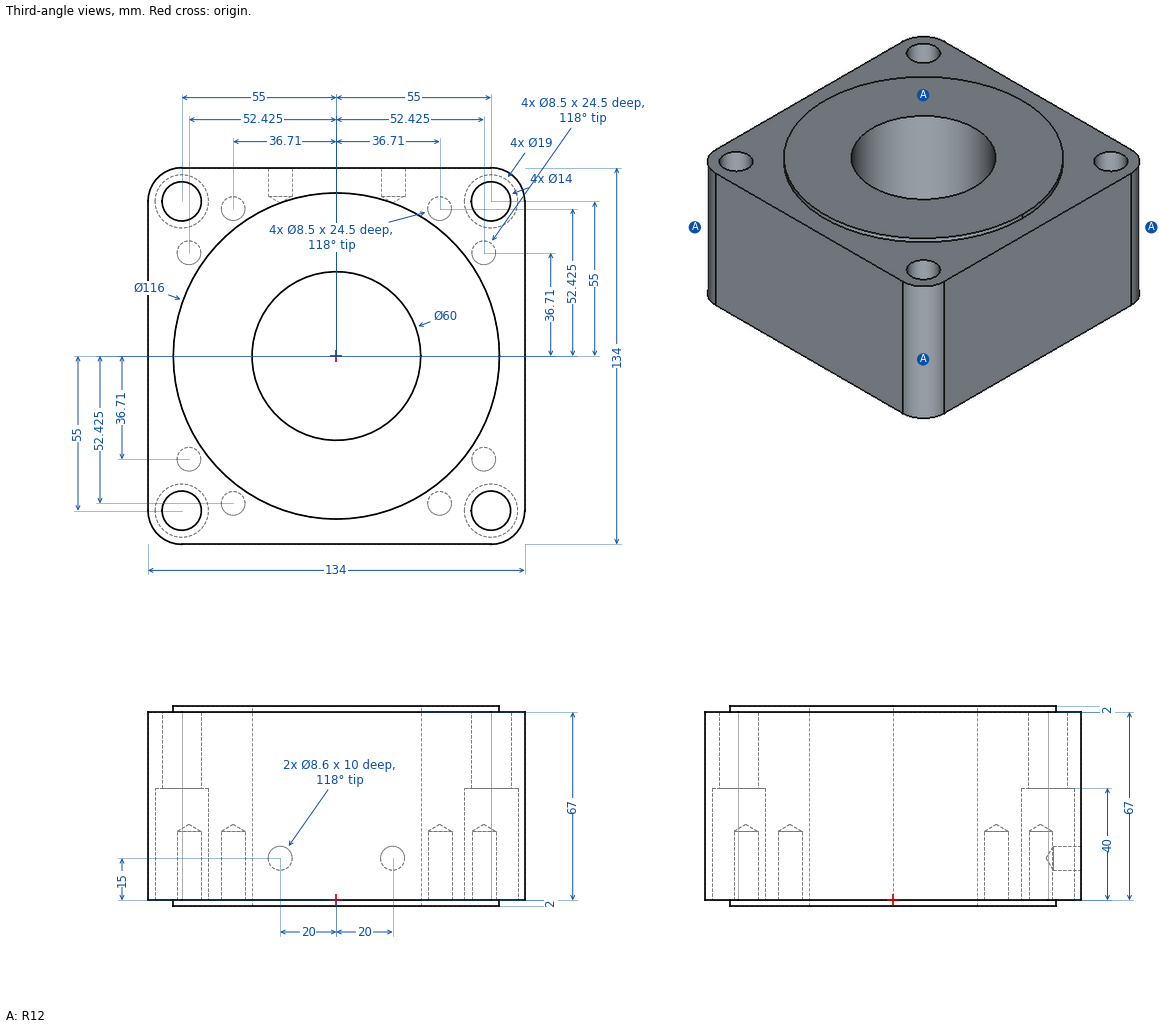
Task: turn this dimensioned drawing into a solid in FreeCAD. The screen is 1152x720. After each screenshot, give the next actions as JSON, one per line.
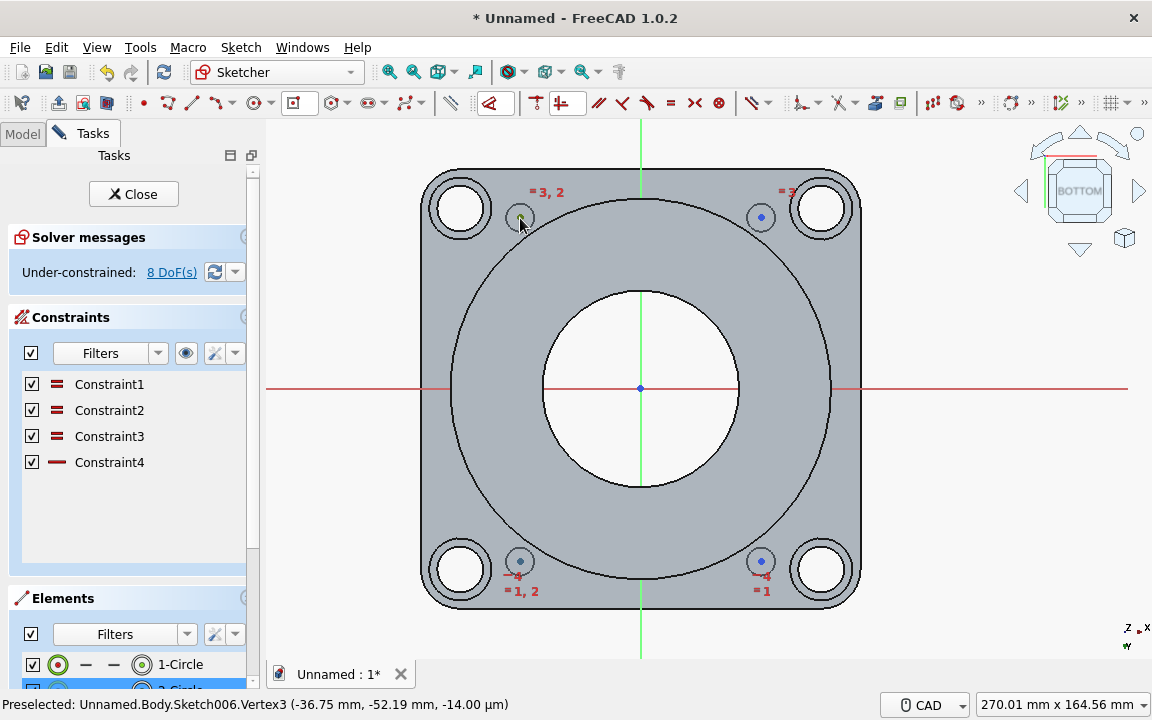
{"action": "key", "text": "v"}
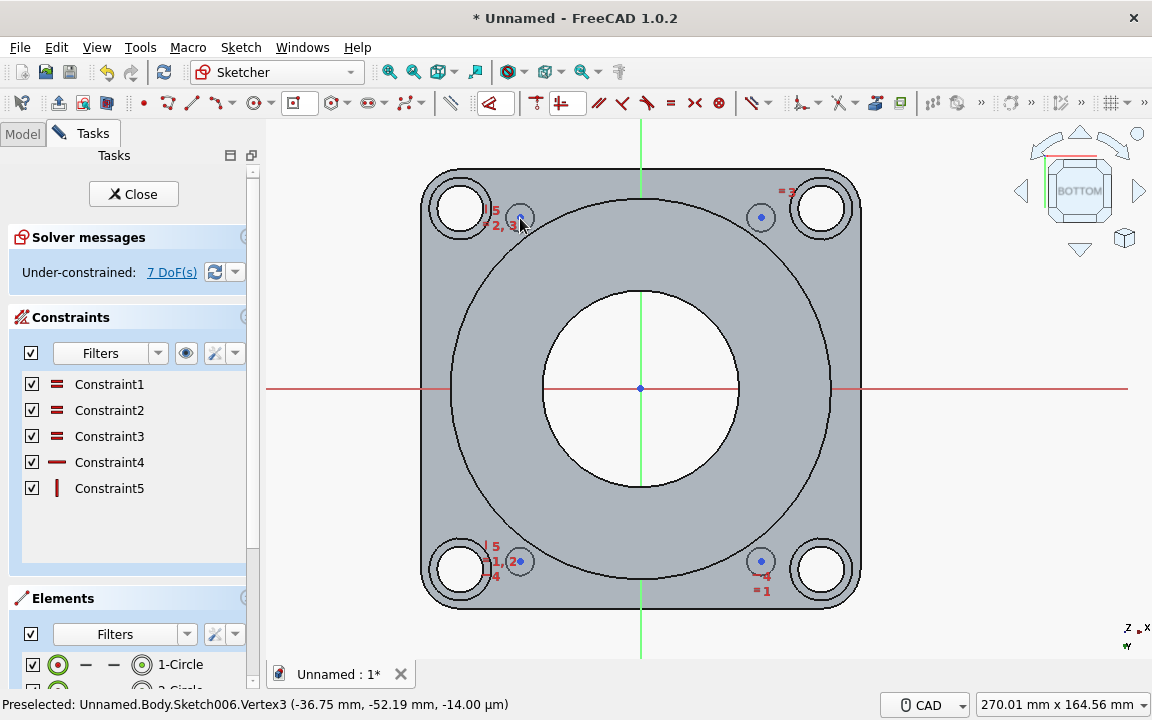
{"action": "left_click", "coordinate": [761, 562]}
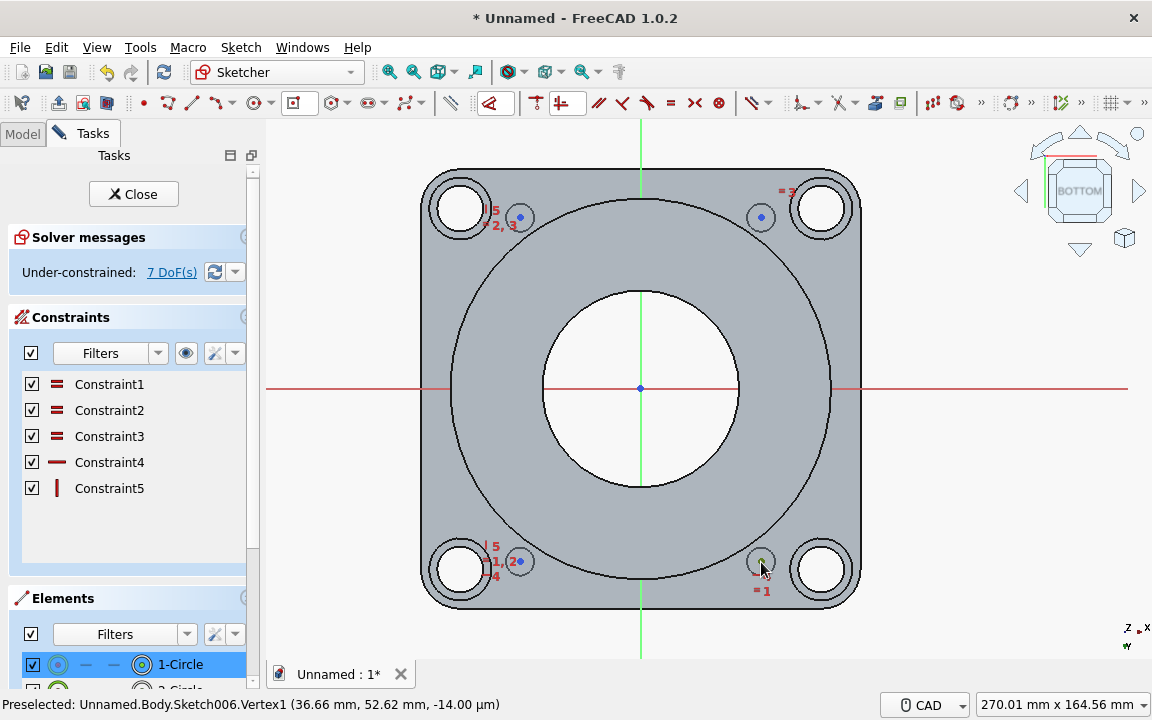
{"action": "left_click", "coordinate": [761, 218]}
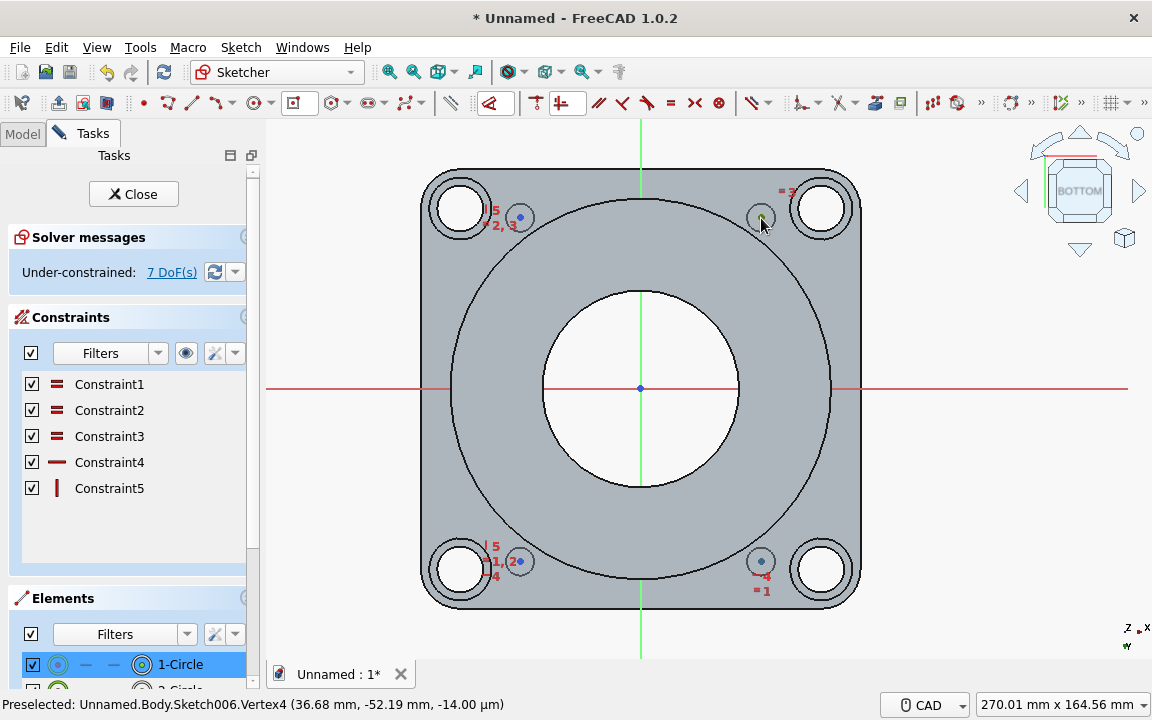
{"action": "key", "text": "v"}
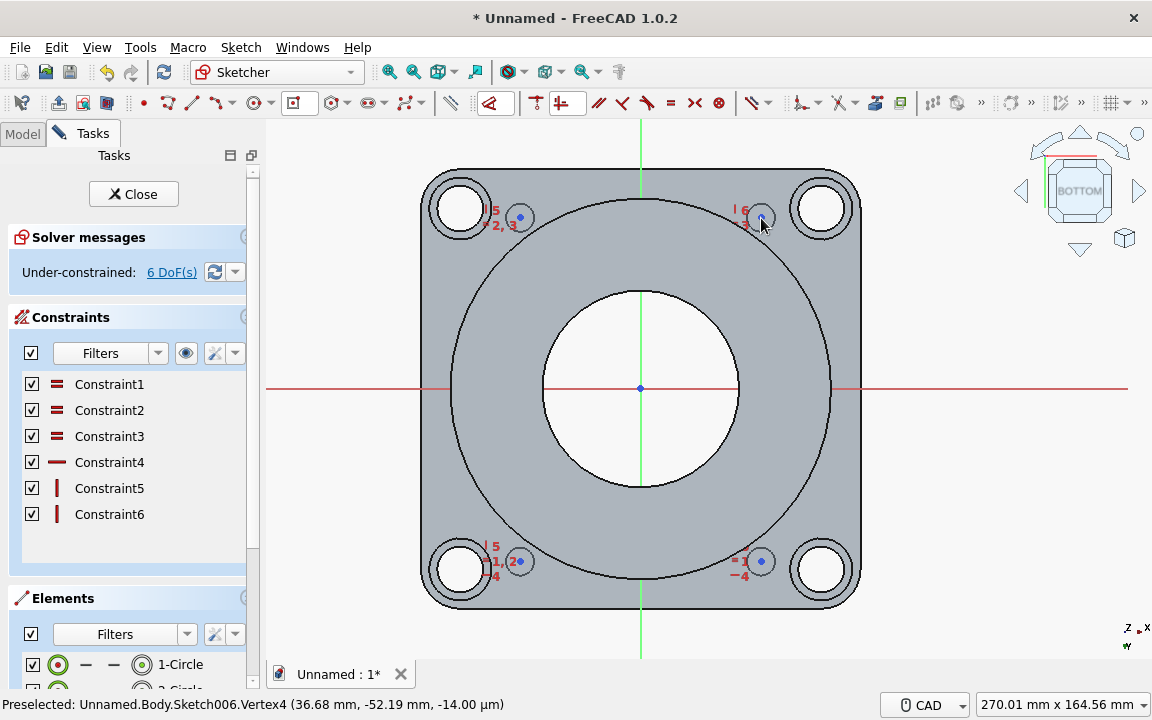
{"action": "left_click", "coordinate": [520, 218]}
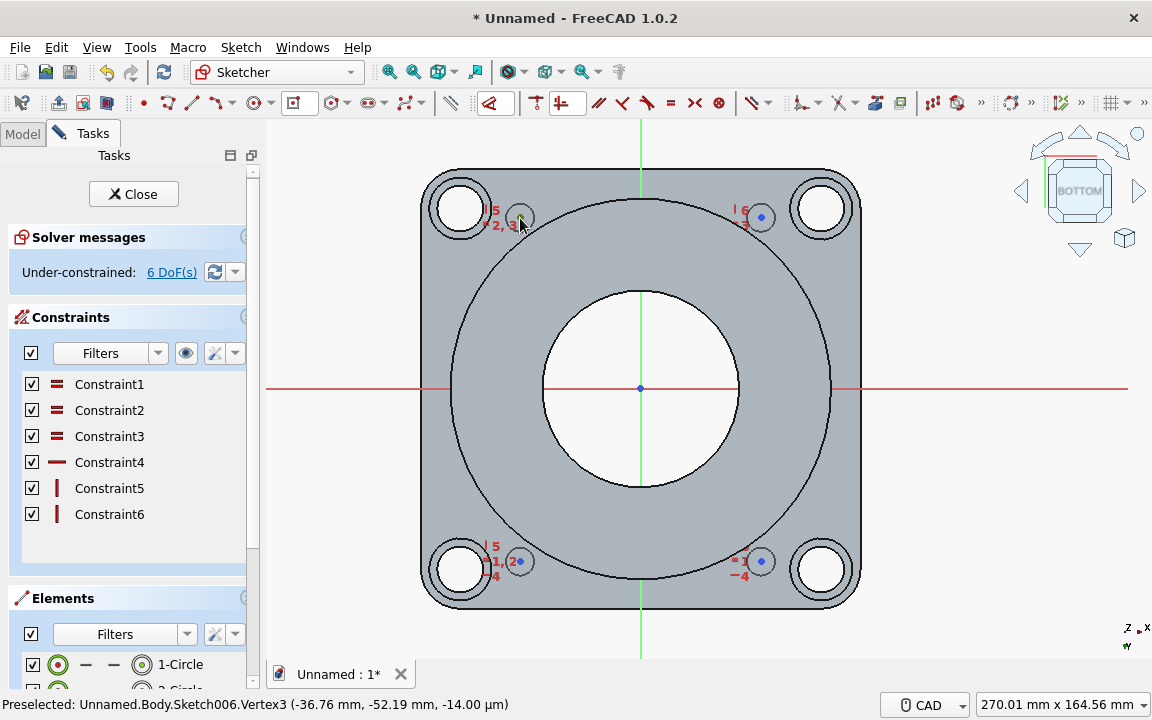
{"action": "left_click", "coordinate": [761, 218]}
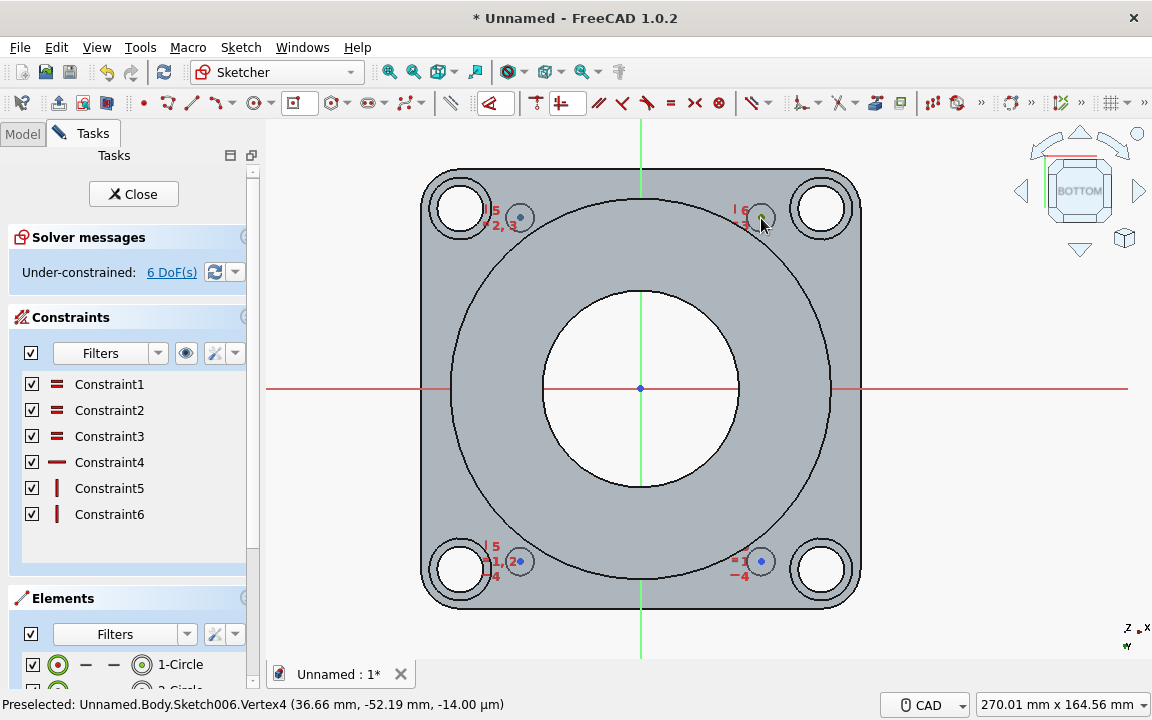
{"action": "key", "text": "h"}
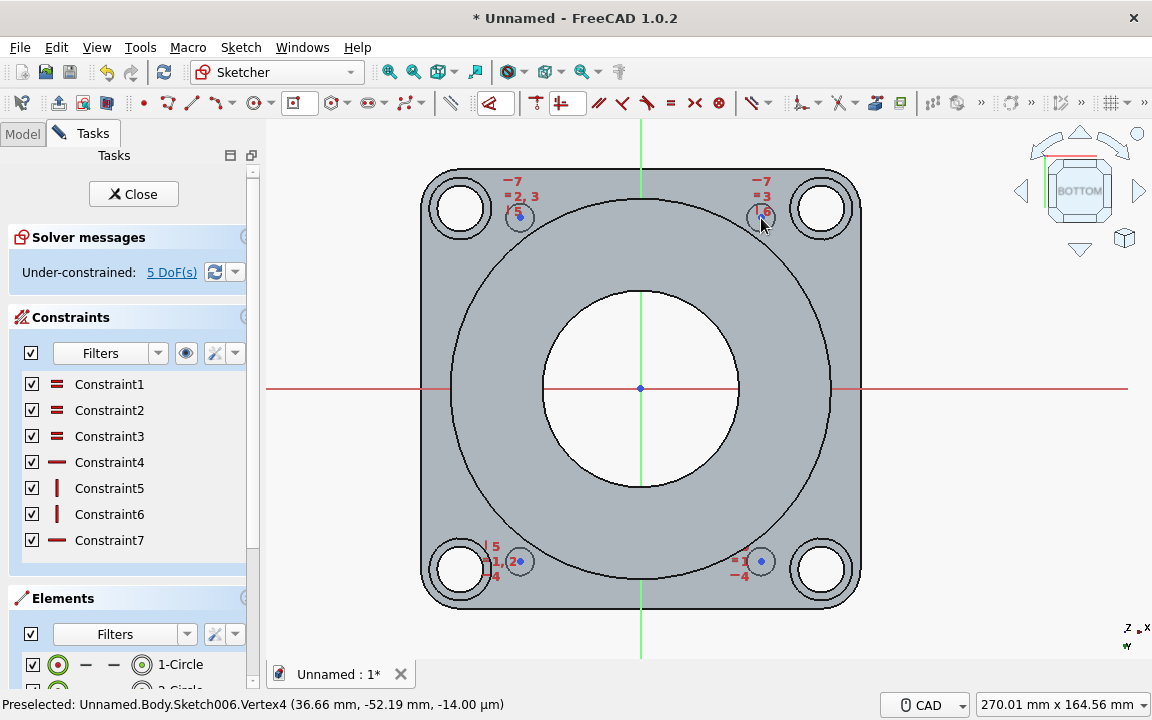
{"action": "scroll", "coordinate": [771, 552], "scroll_direction": "up", "scroll_amount": 2}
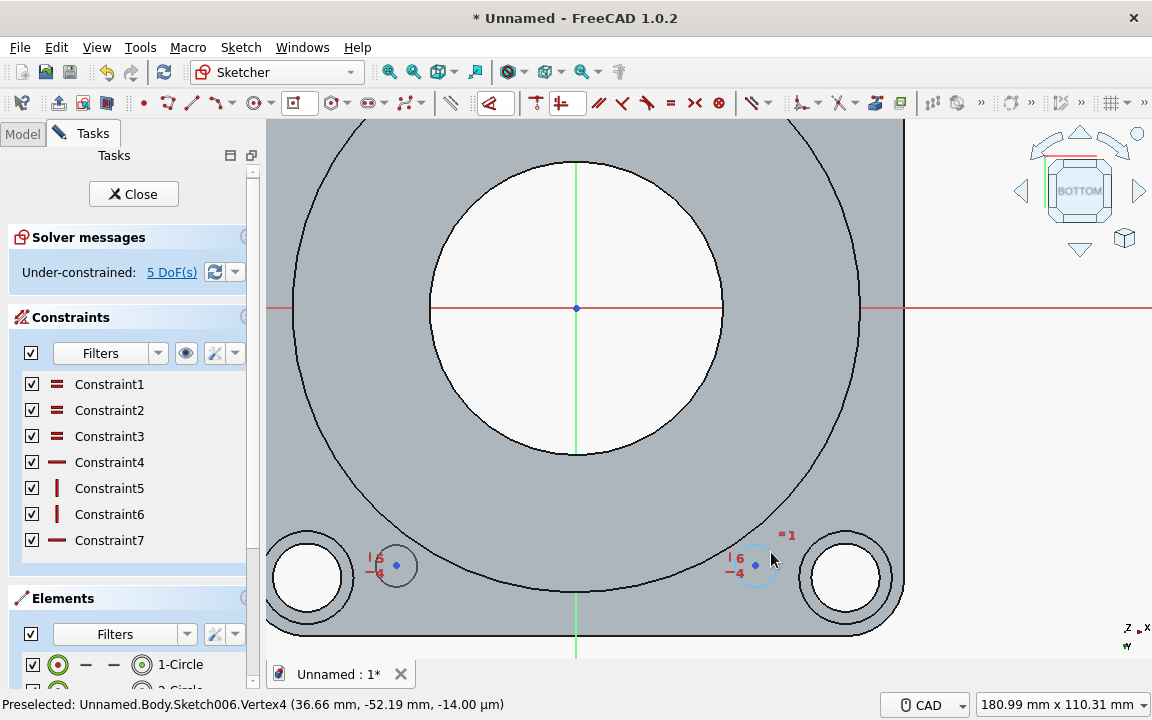
{"action": "left_click", "coordinate": [771, 551]}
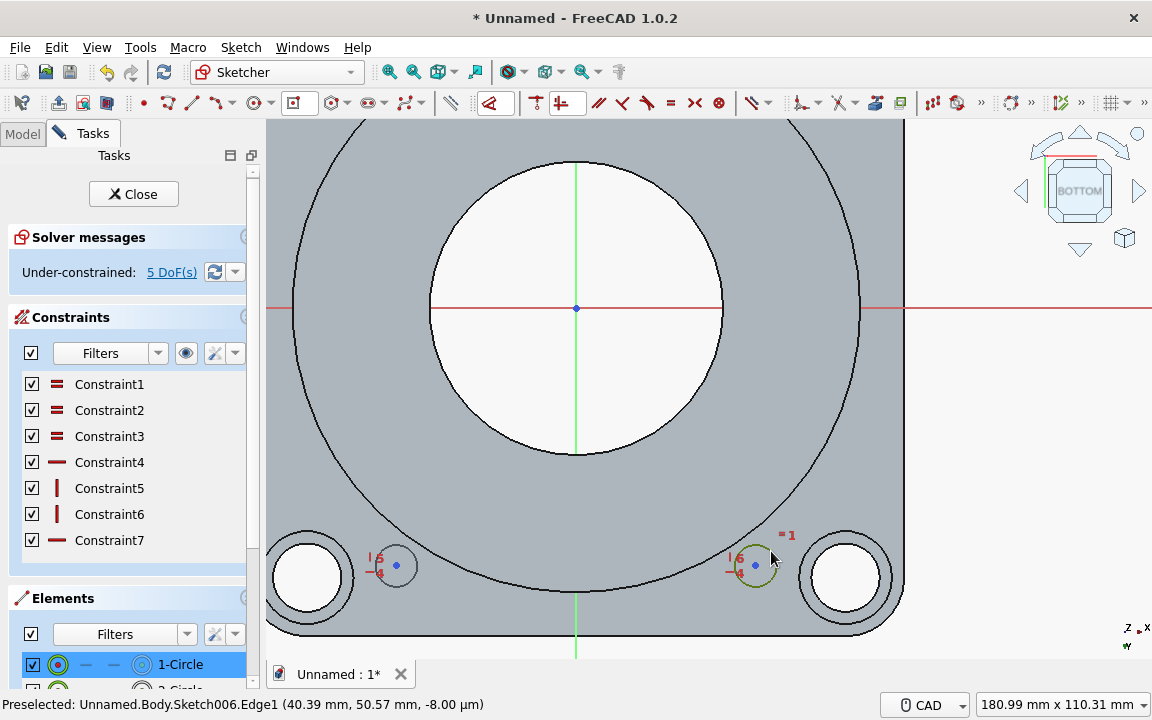
{"action": "left_click", "coordinate": [508, 104]}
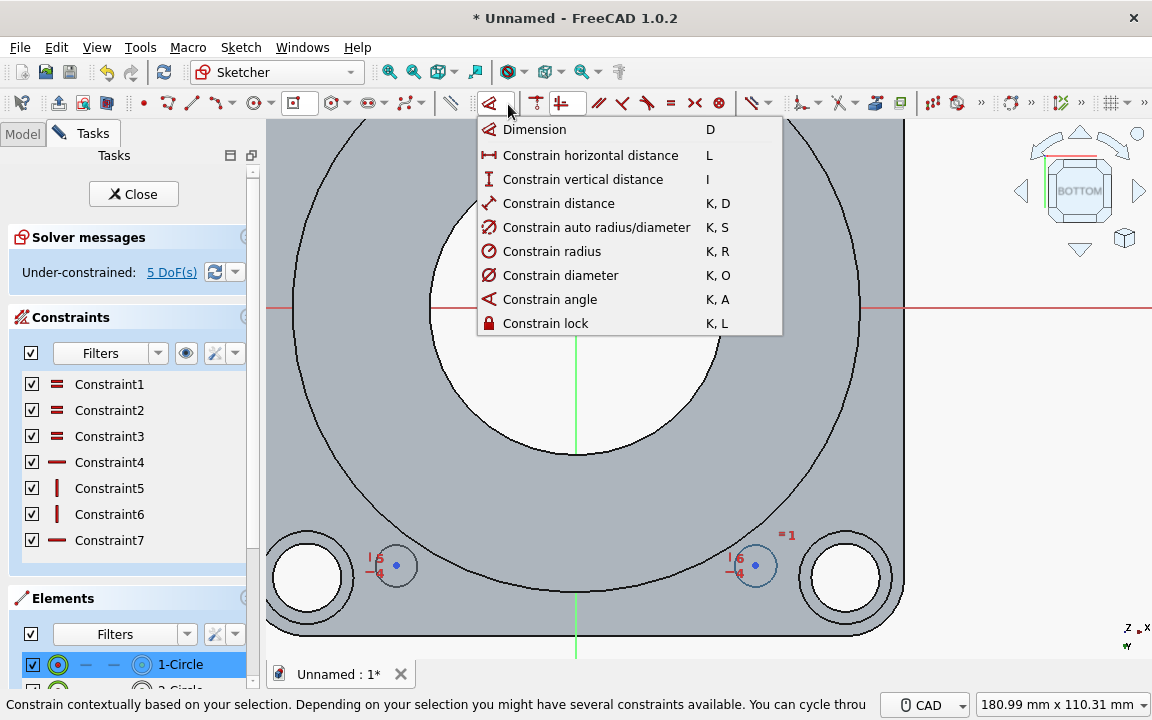
{"action": "left_click", "coordinate": [630, 275]}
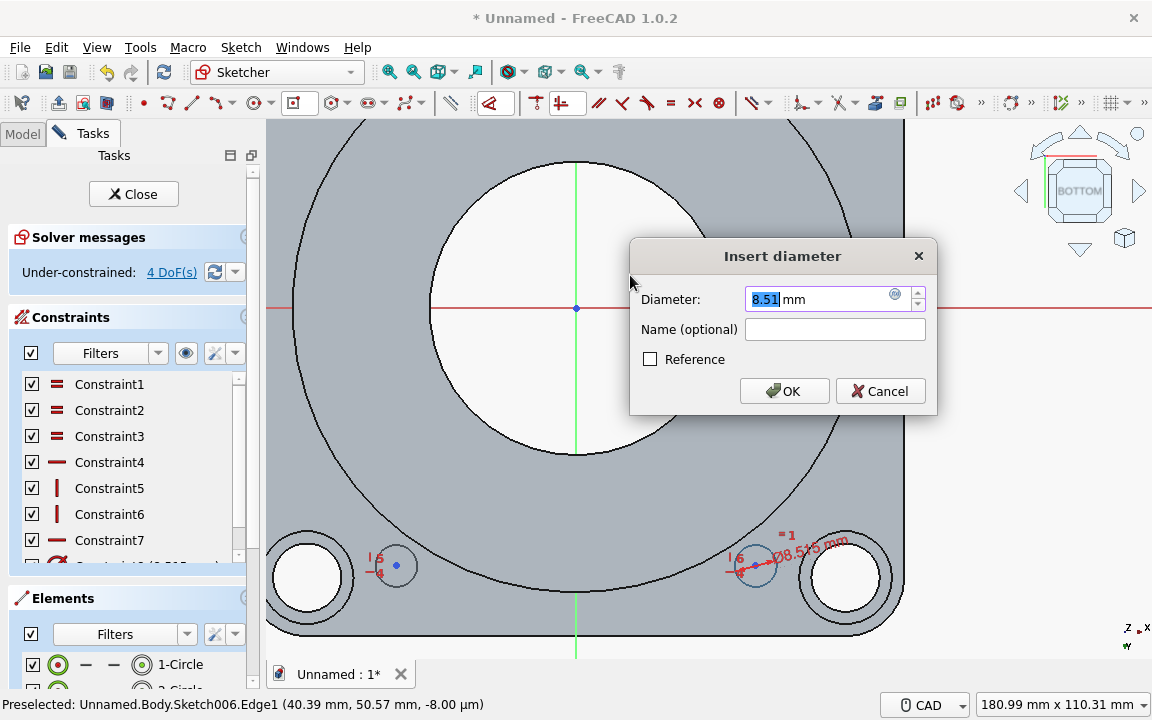
{"action": "type", "text": "8.5"}
{"action": "key", "text": "Return"}